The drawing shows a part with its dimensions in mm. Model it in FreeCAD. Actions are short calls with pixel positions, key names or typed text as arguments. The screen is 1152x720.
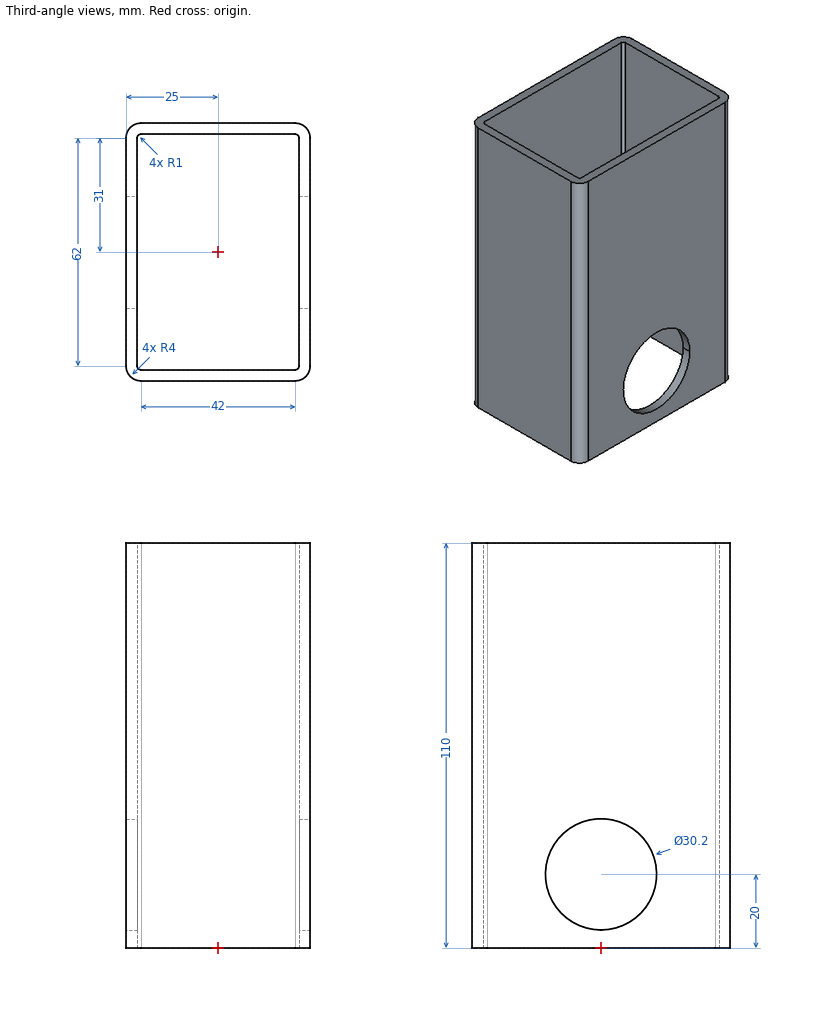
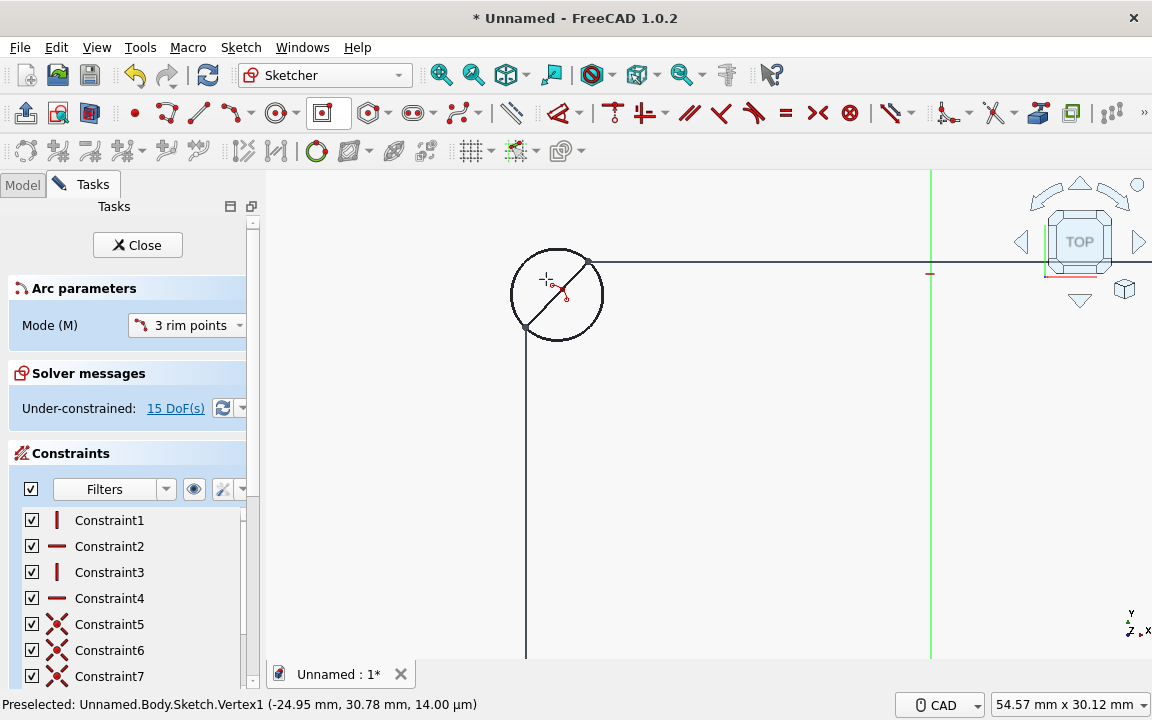
click(544, 278)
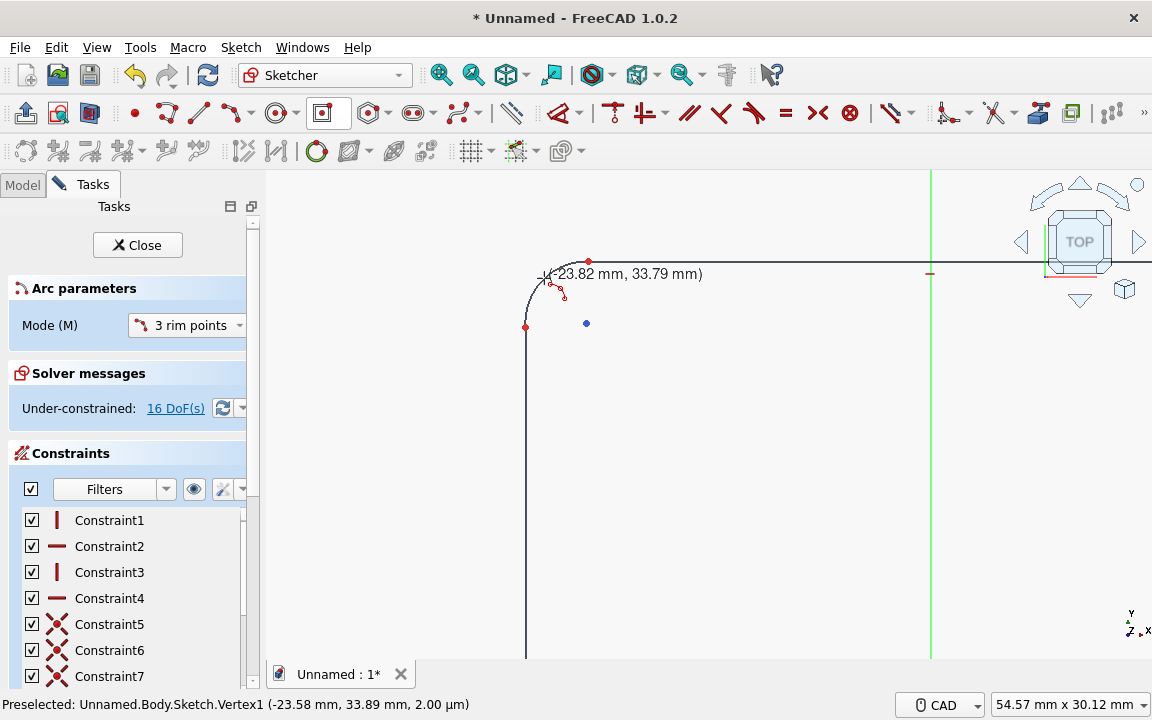
key(g)
key(l)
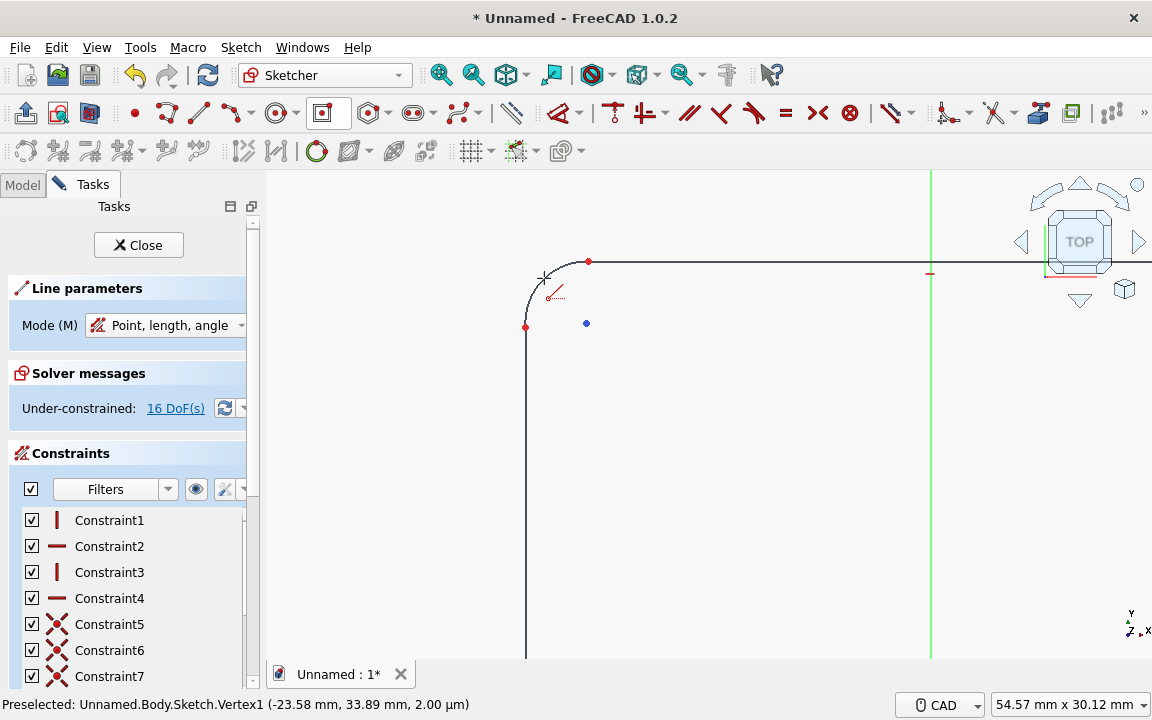
scroll(546, 279, down, 7)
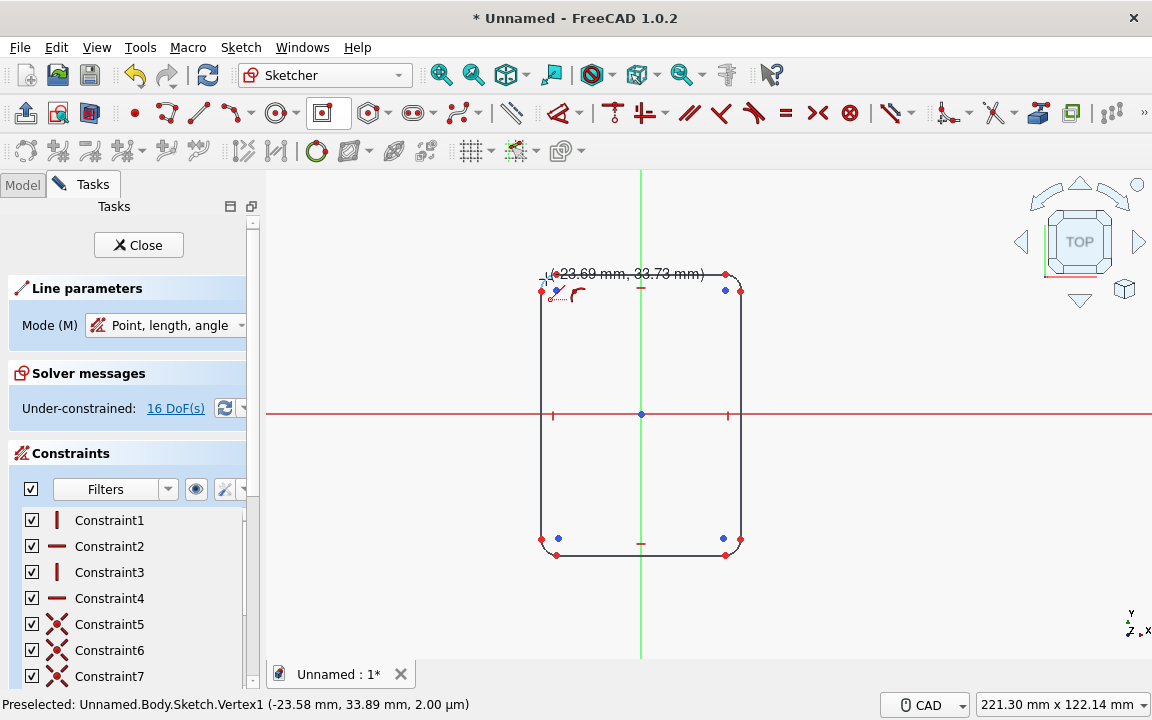
scroll(553, 539, up, 7)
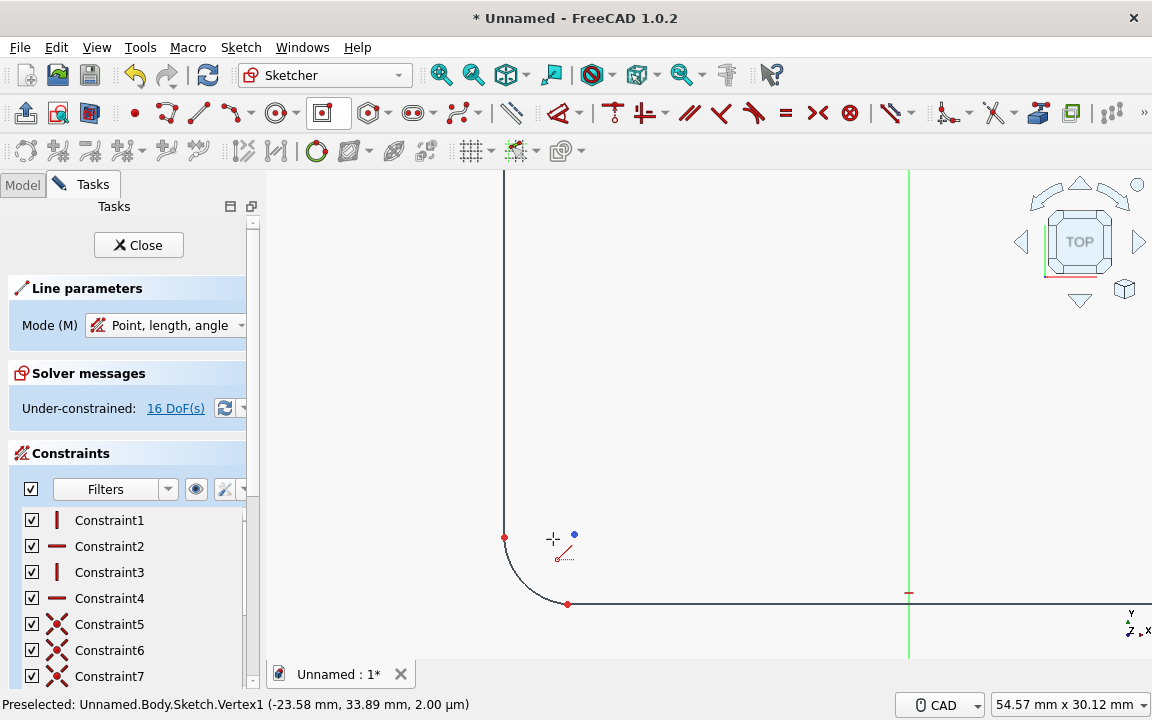
click(552, 535)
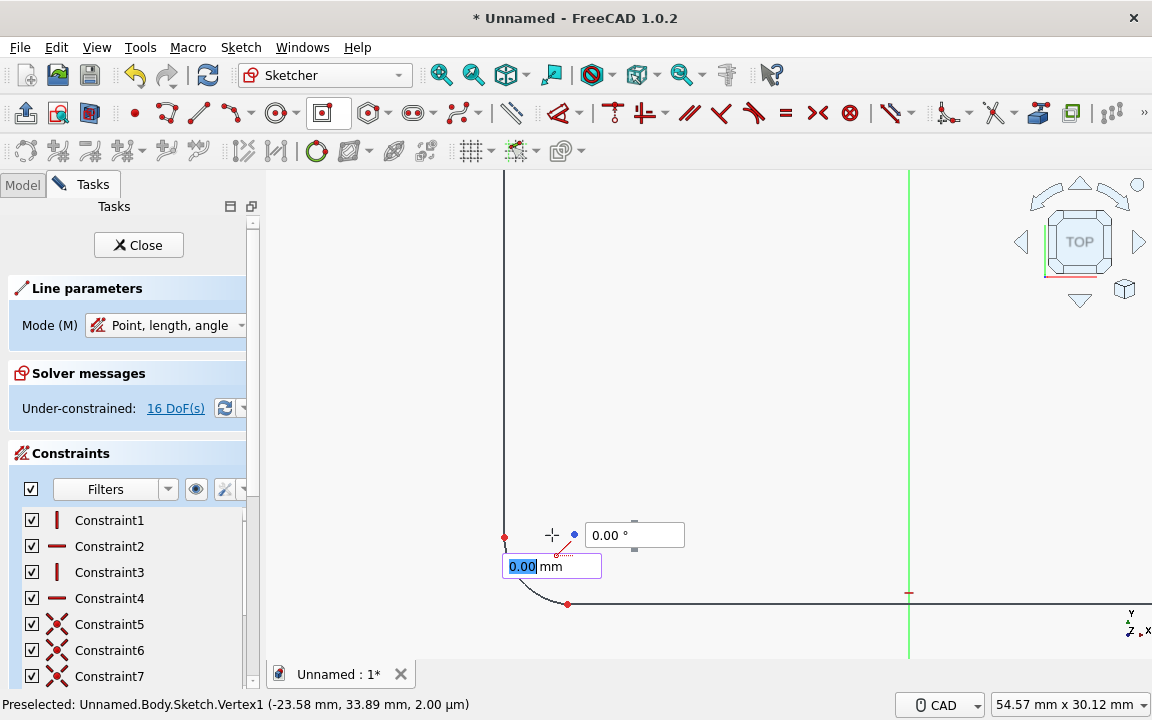
scroll(553, 540, down, 7)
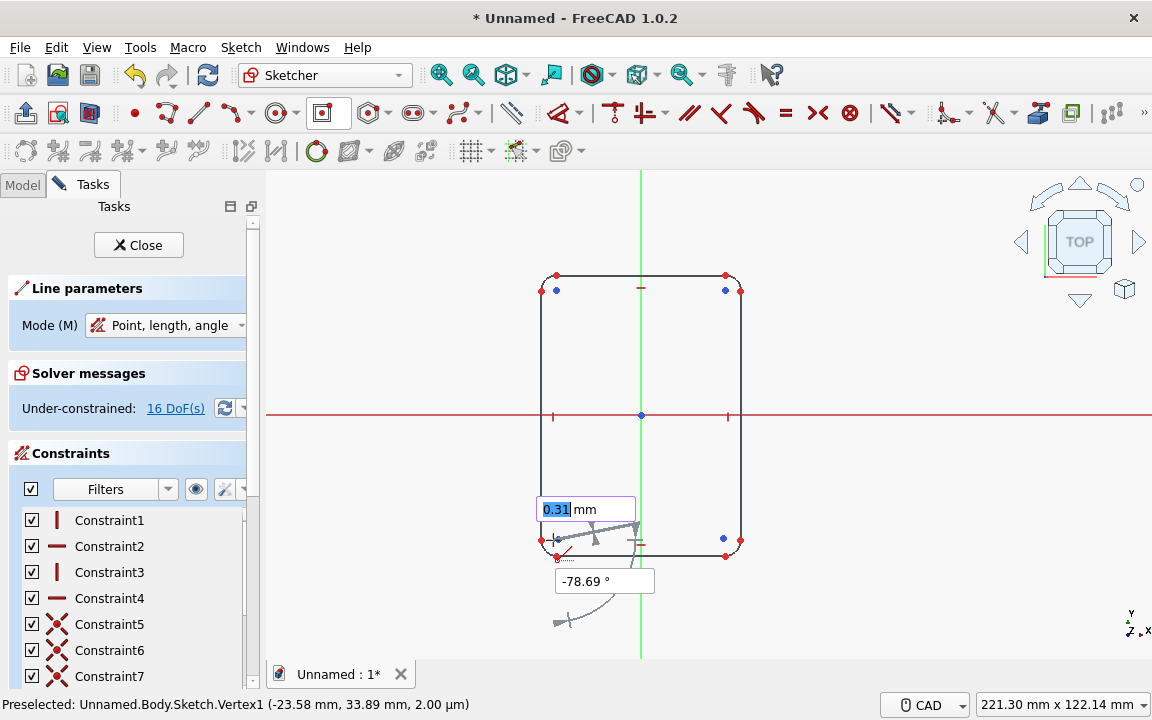
scroll(553, 291, up, 7)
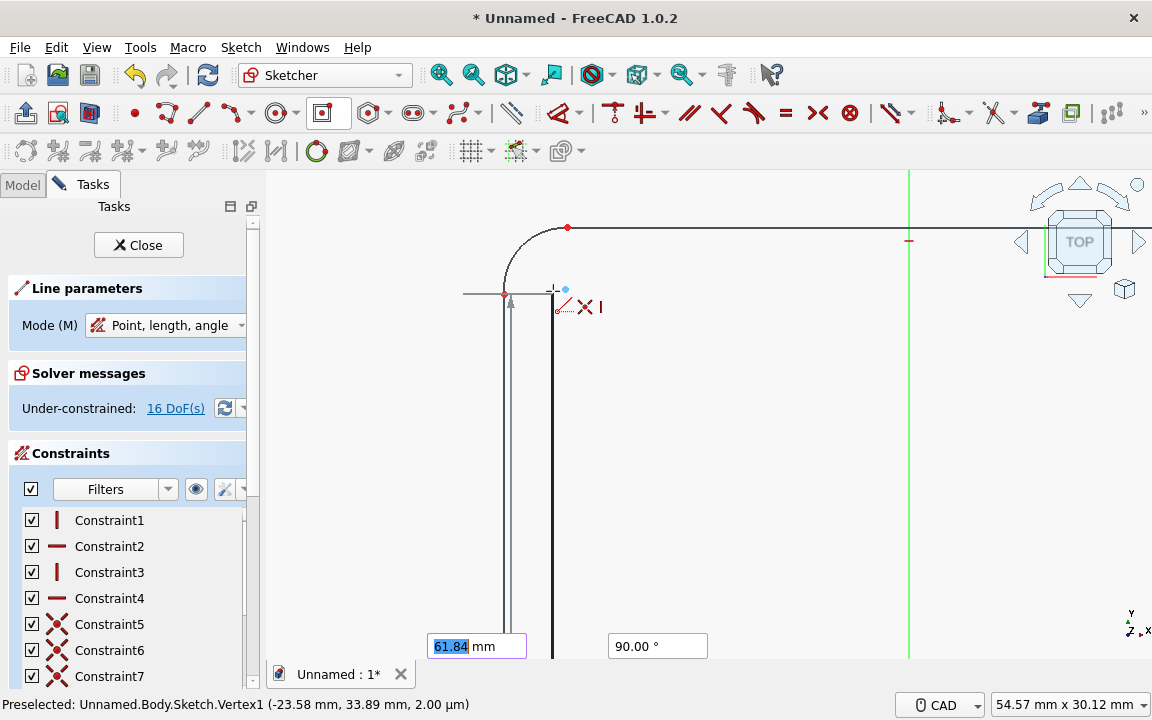
click(552, 291)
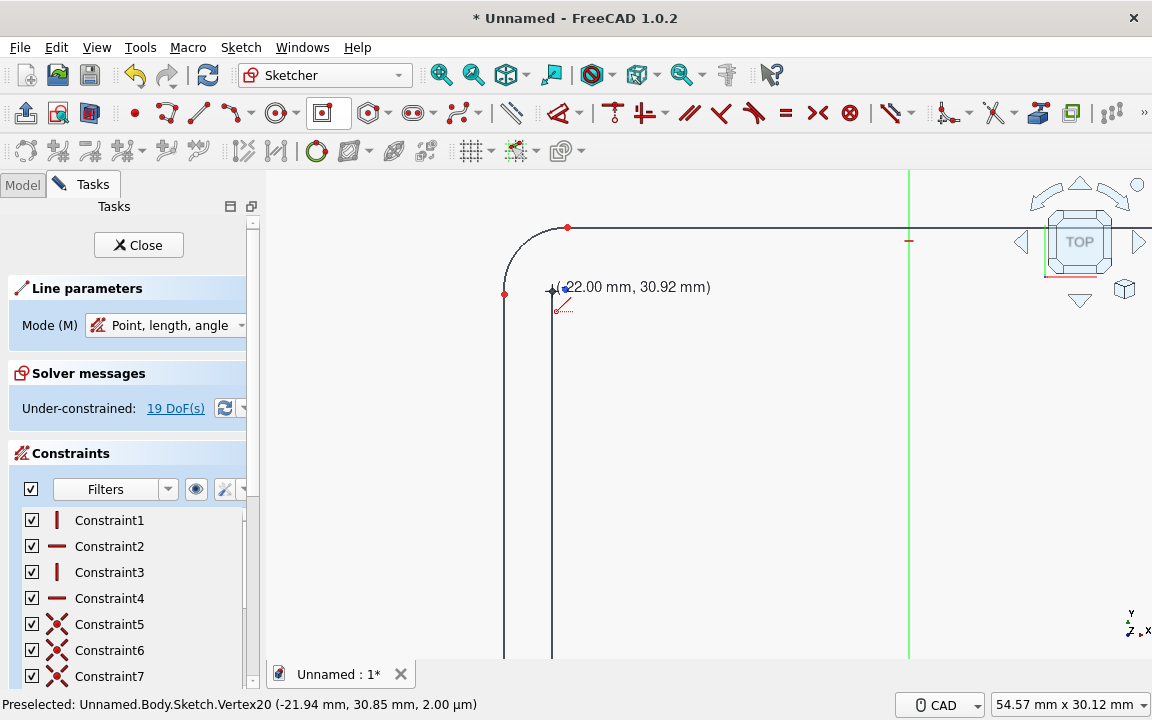
click(568, 274)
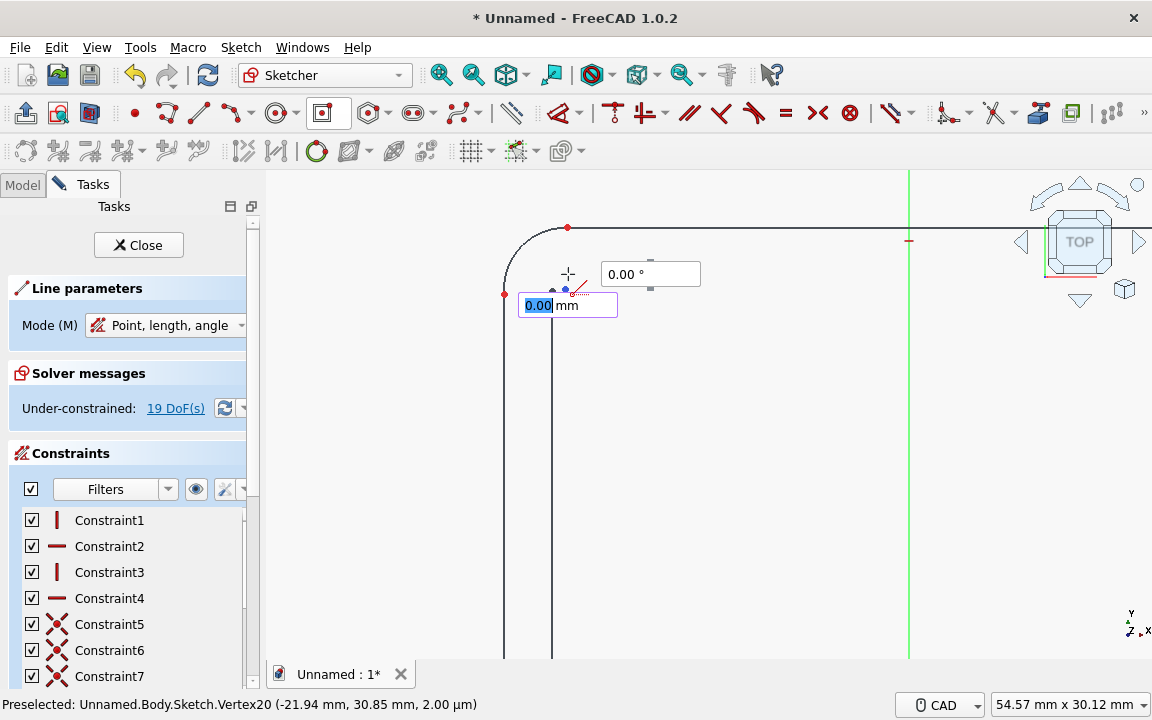
scroll(553, 290, down, 7)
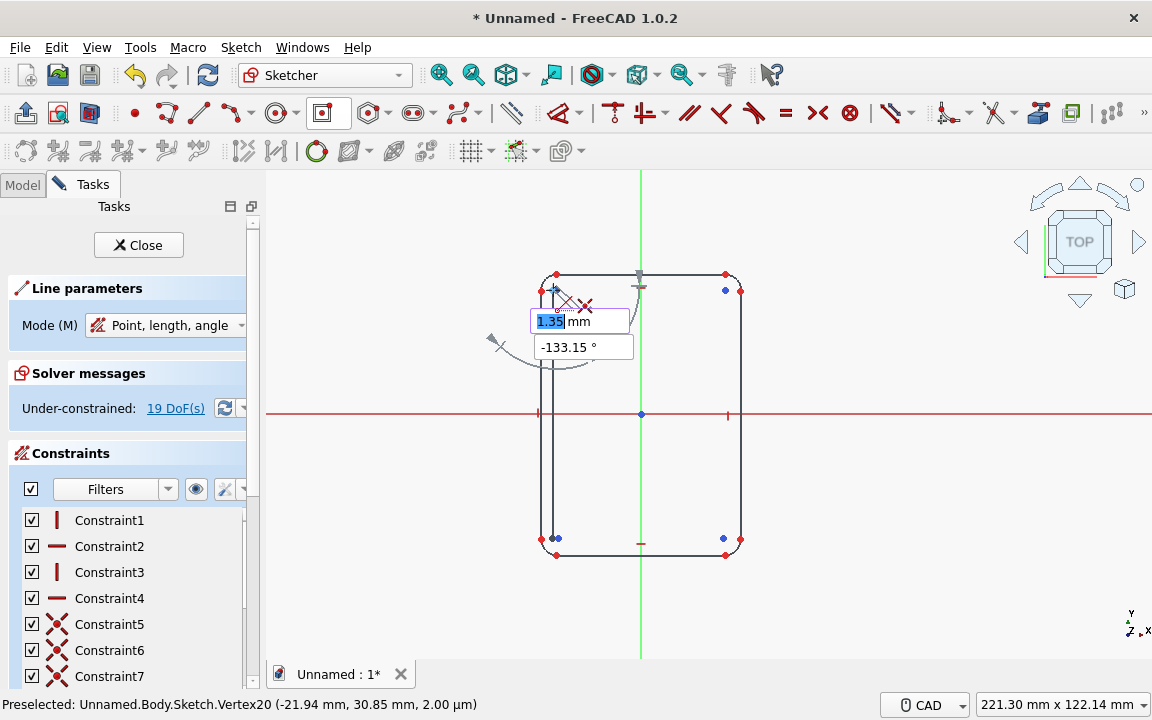
scroll(725, 286, up, 7)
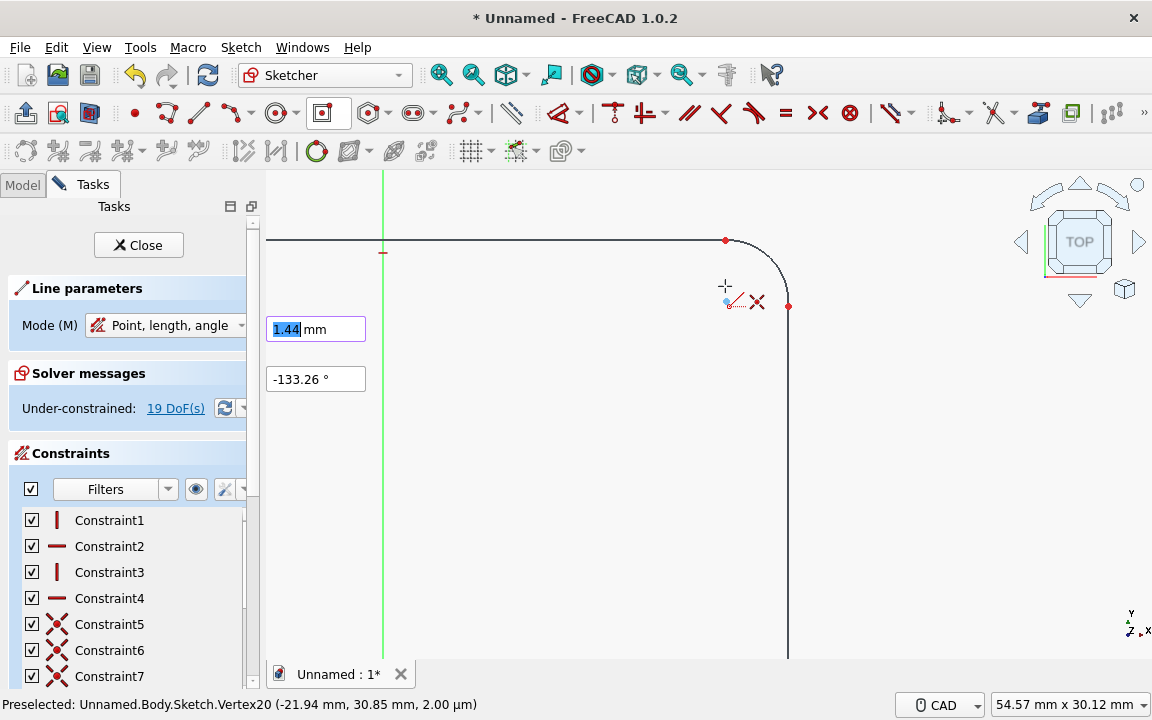
click(724, 286)